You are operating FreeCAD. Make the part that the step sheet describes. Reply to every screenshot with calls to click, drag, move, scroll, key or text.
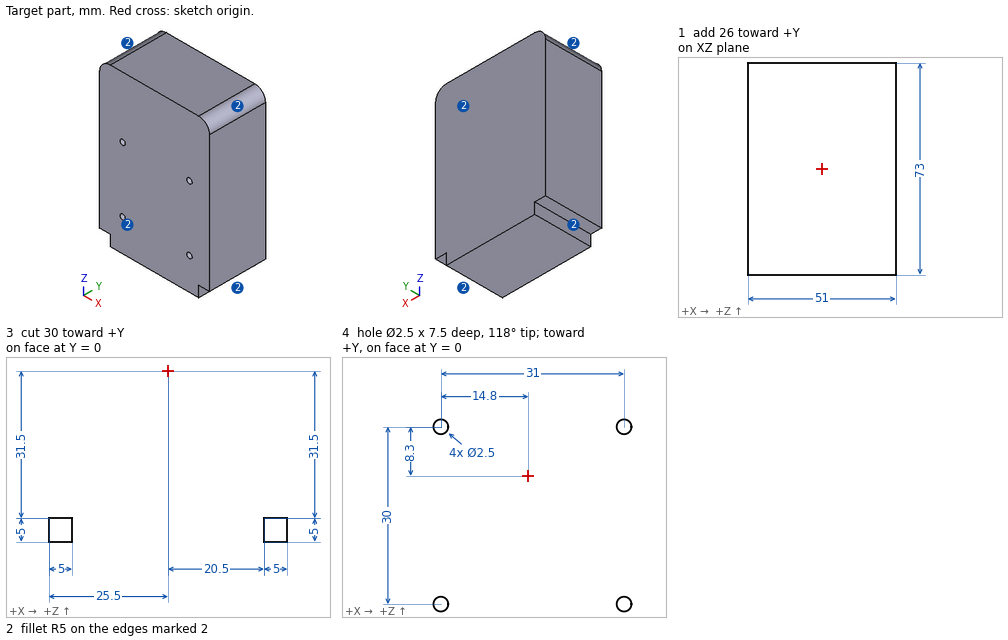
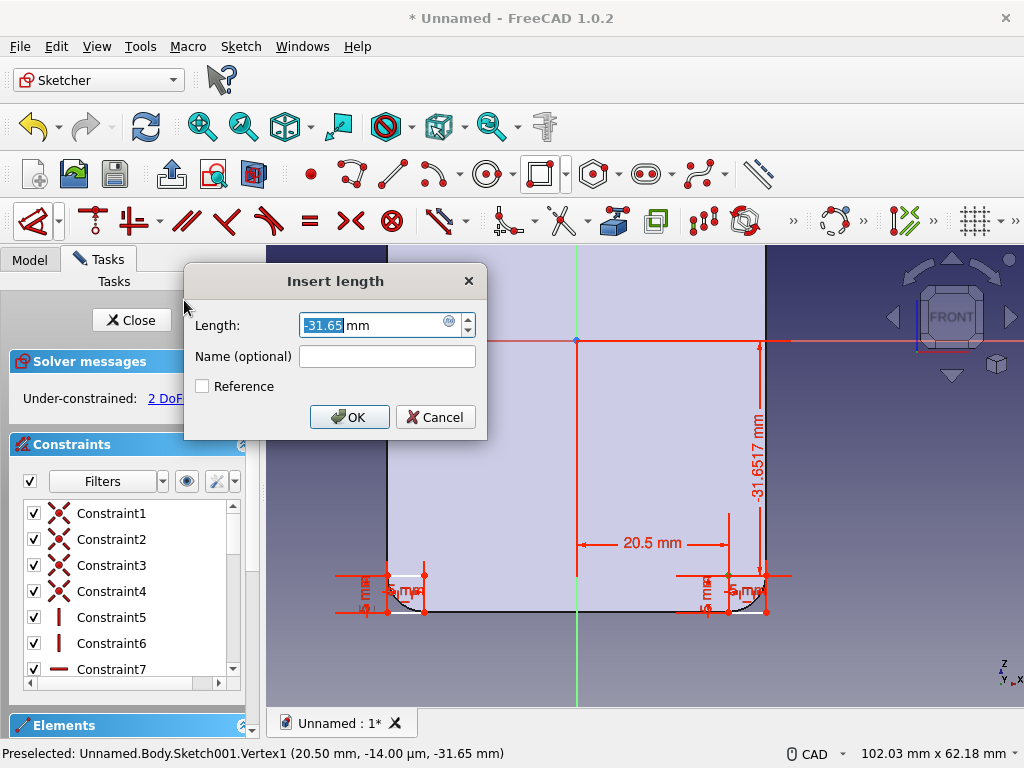
text(-31.5)
key(Return)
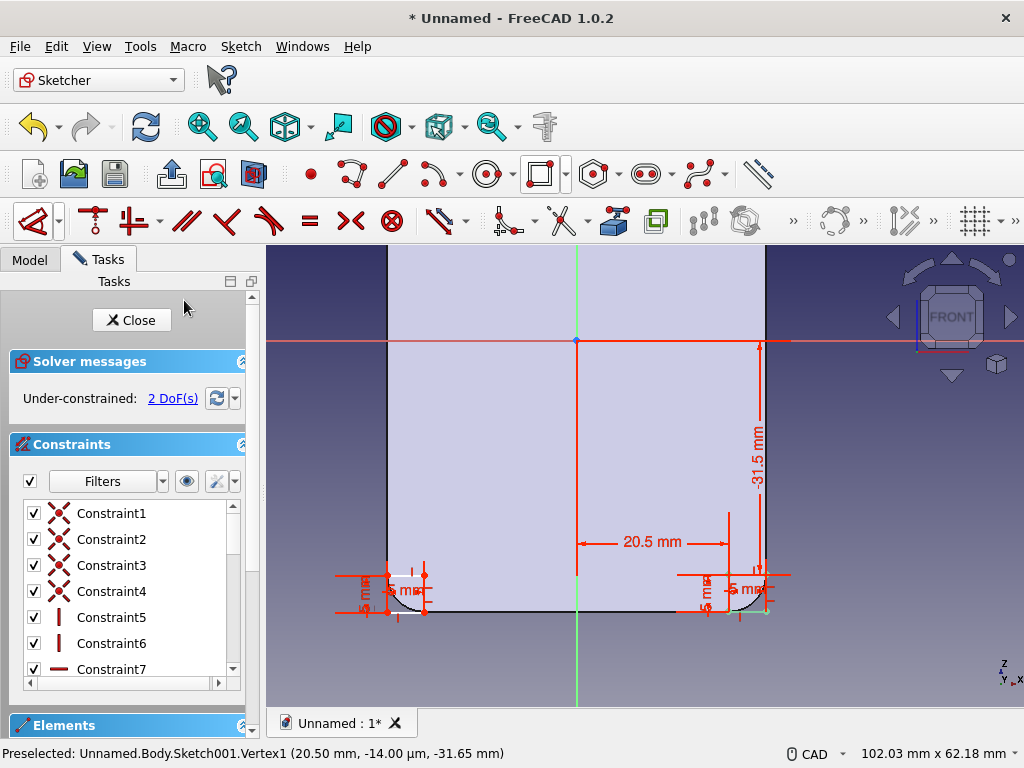
click(387, 576)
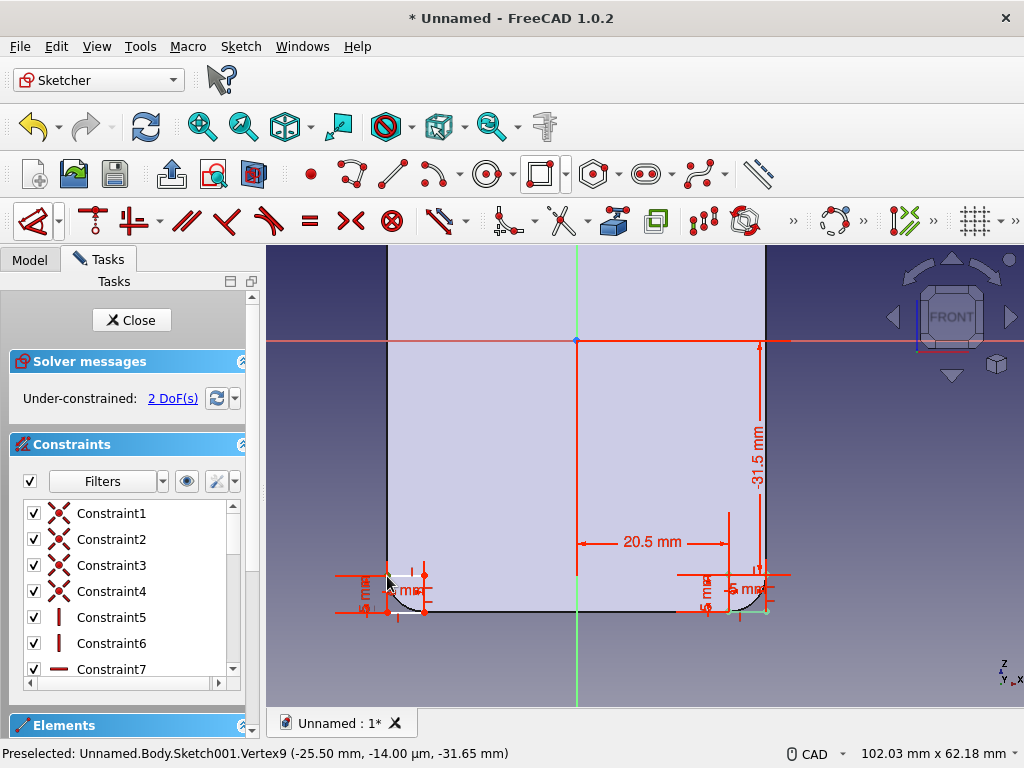
click(58, 222)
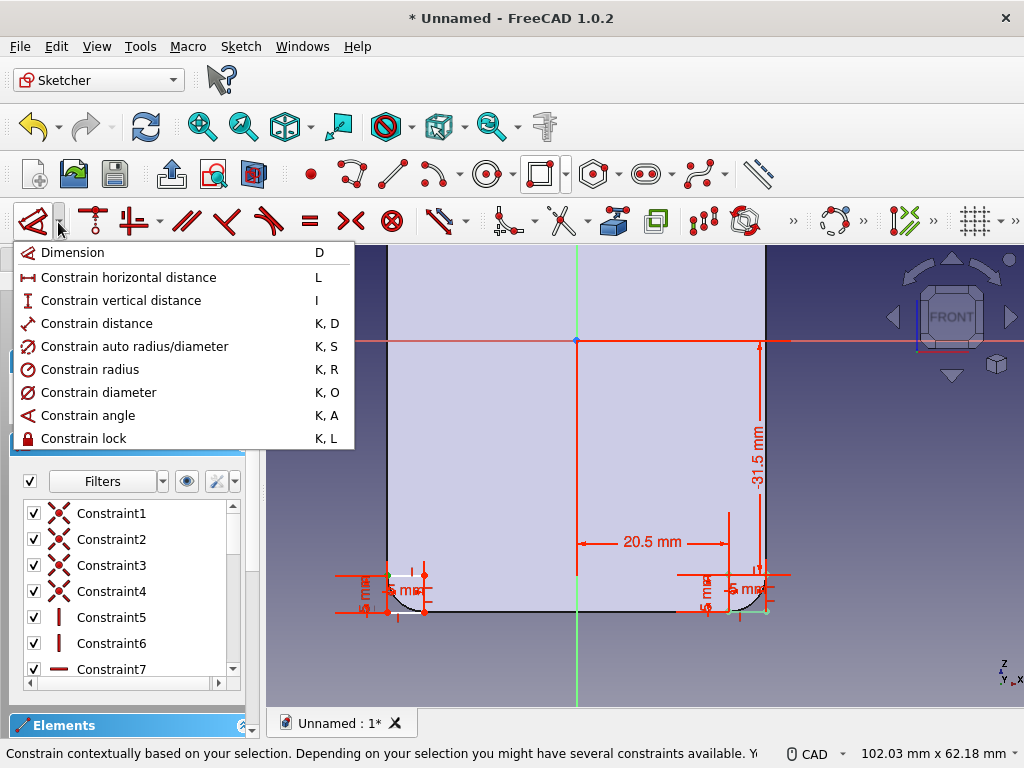
click(184, 278)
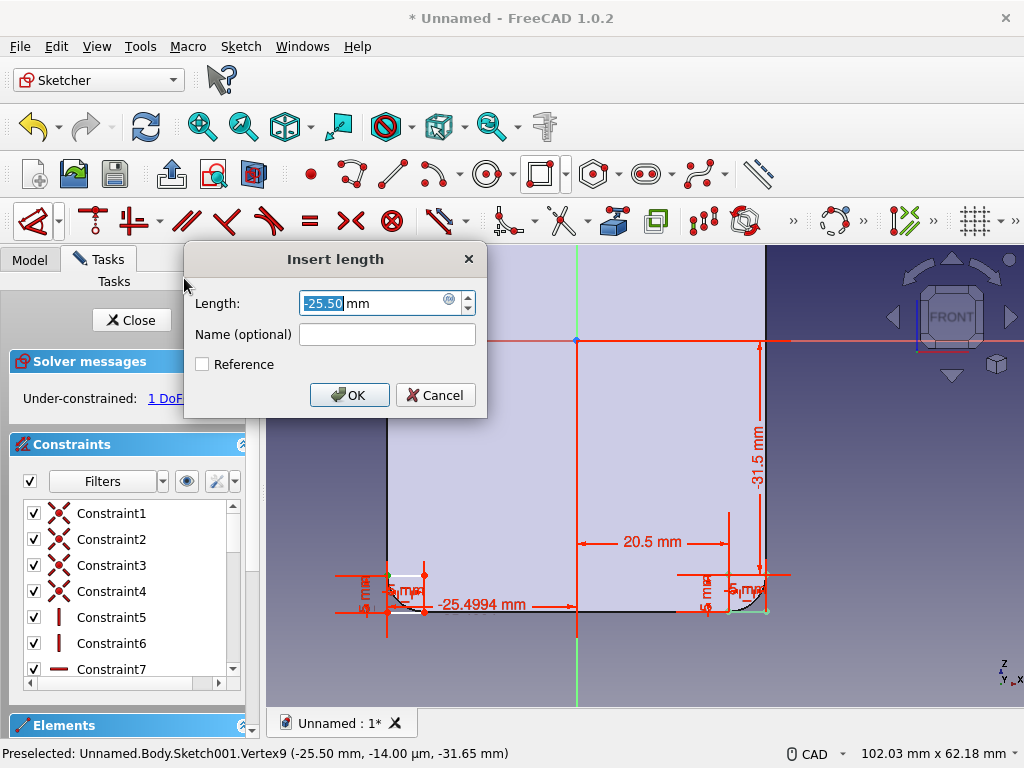
text(-25.5)
key(Return)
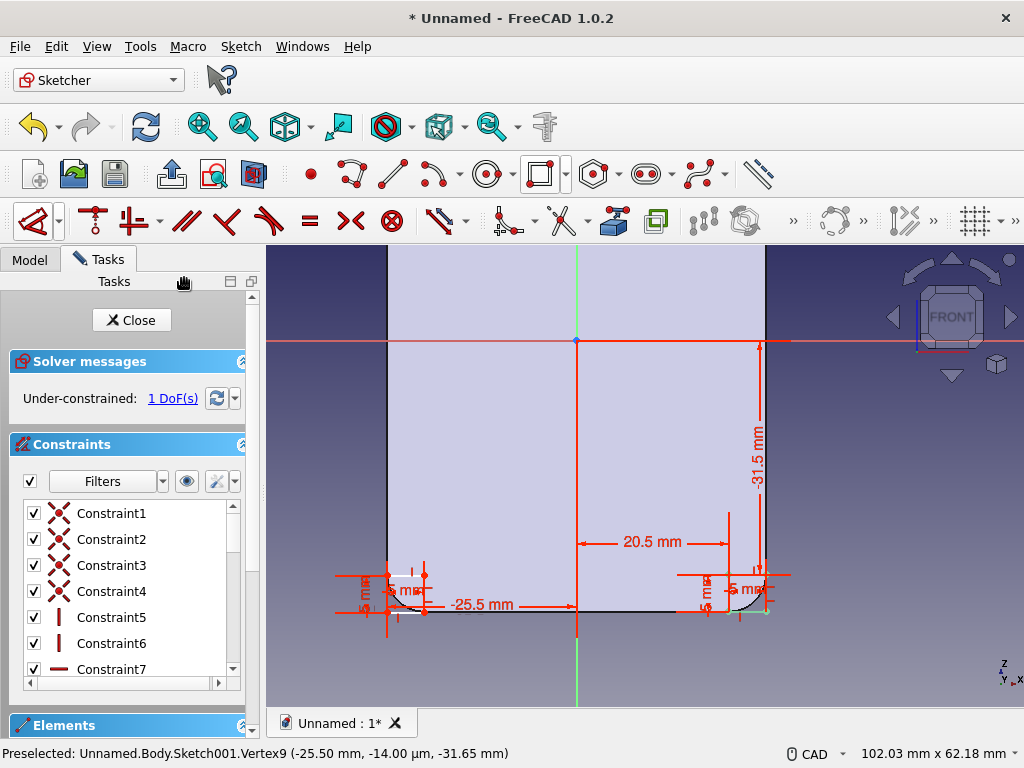
click(387, 576)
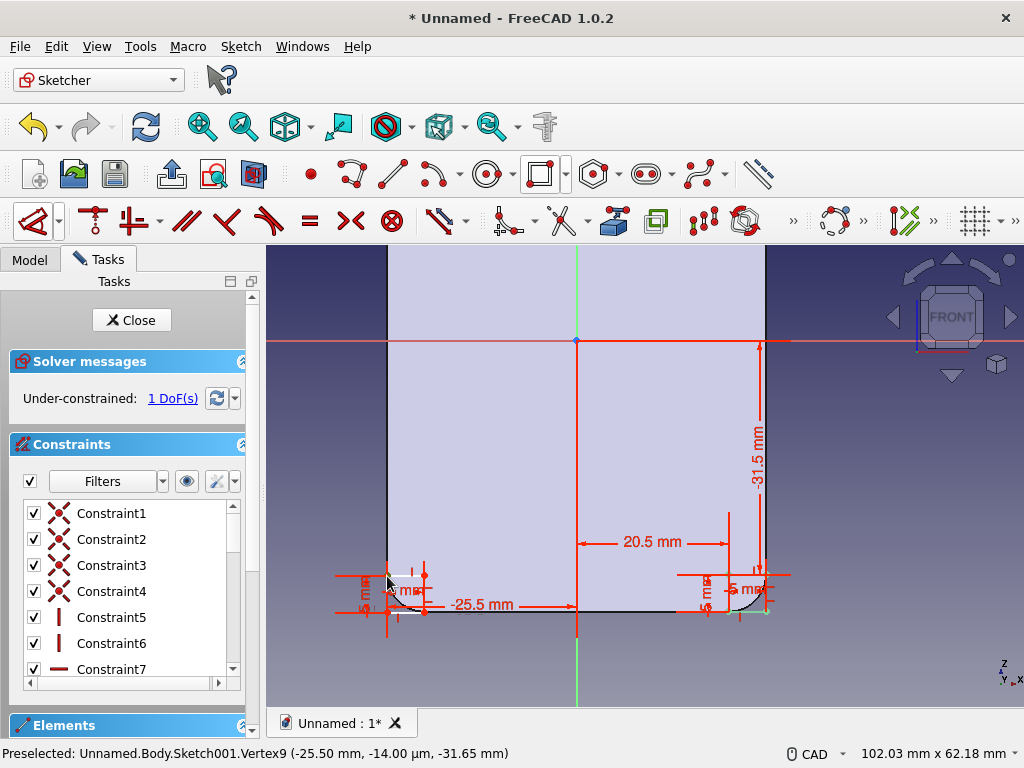
key(i)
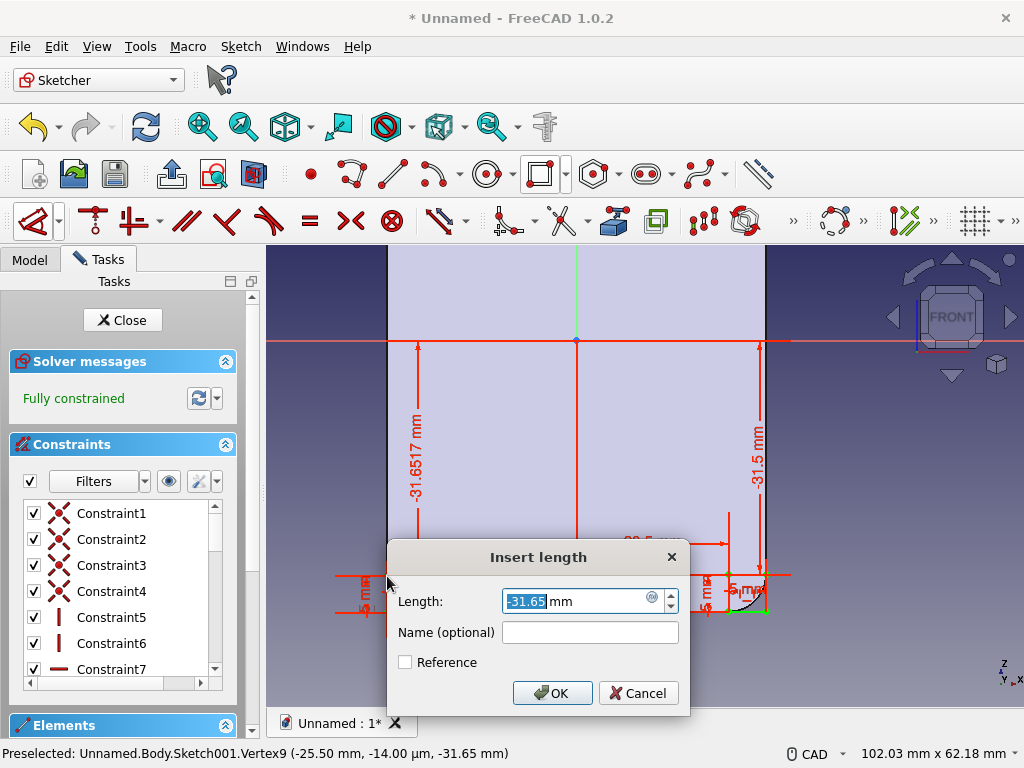
text(-31.5)
key(Return)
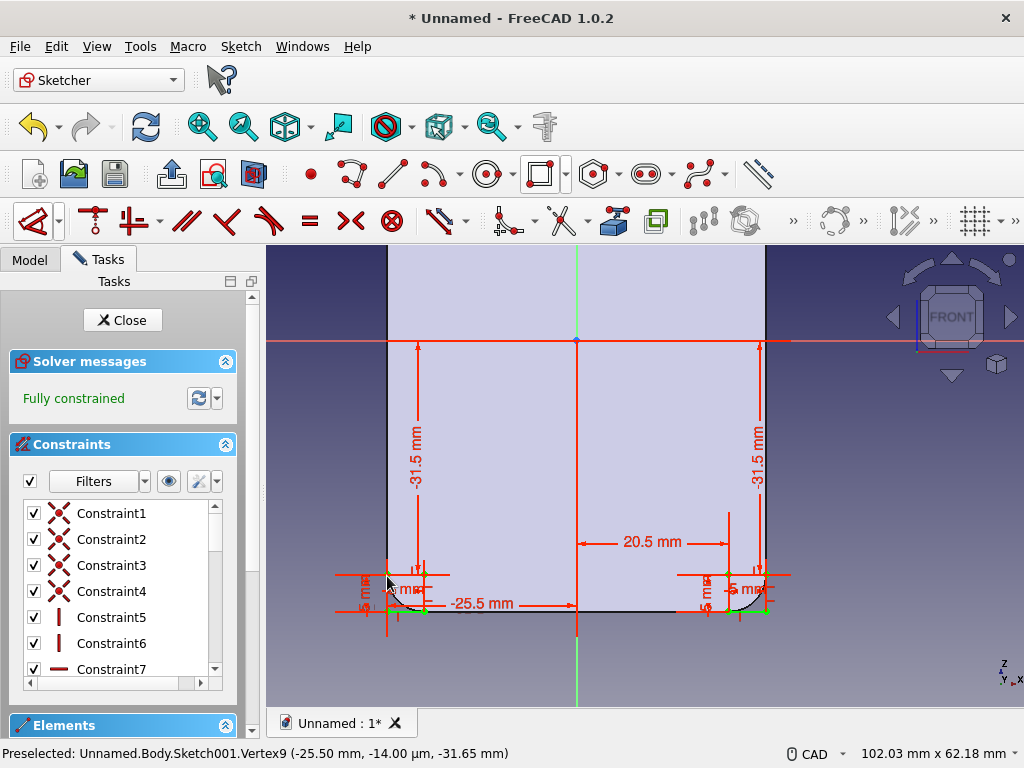
click(123, 320)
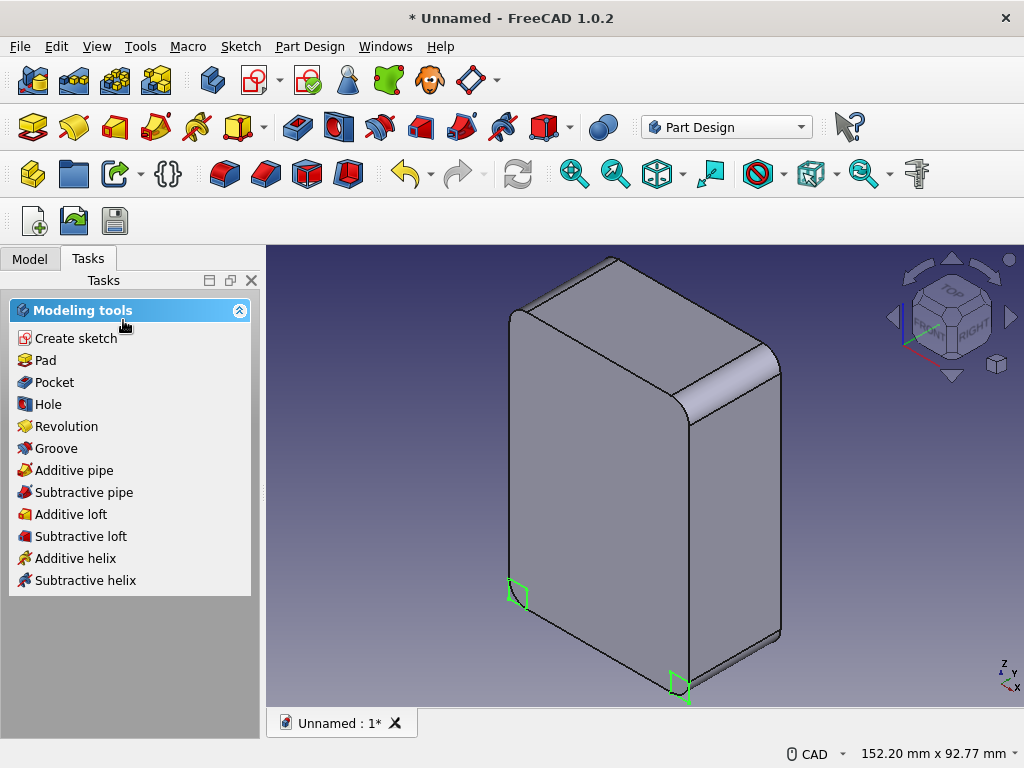
click(298, 128)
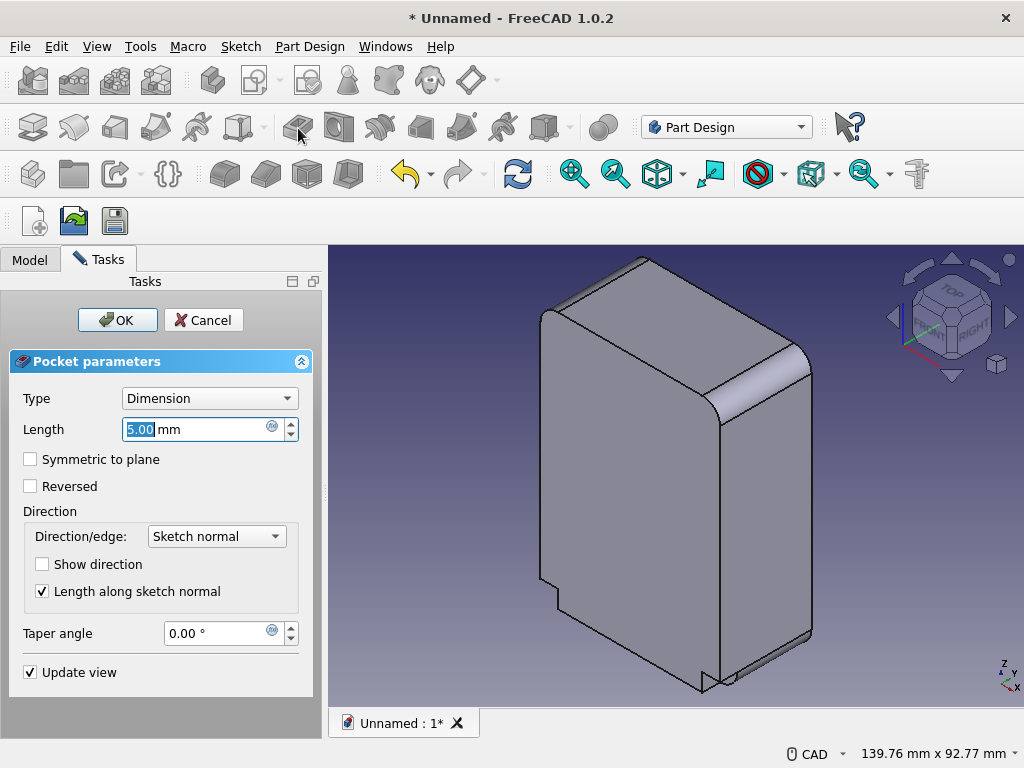
text(30)
key(Tab)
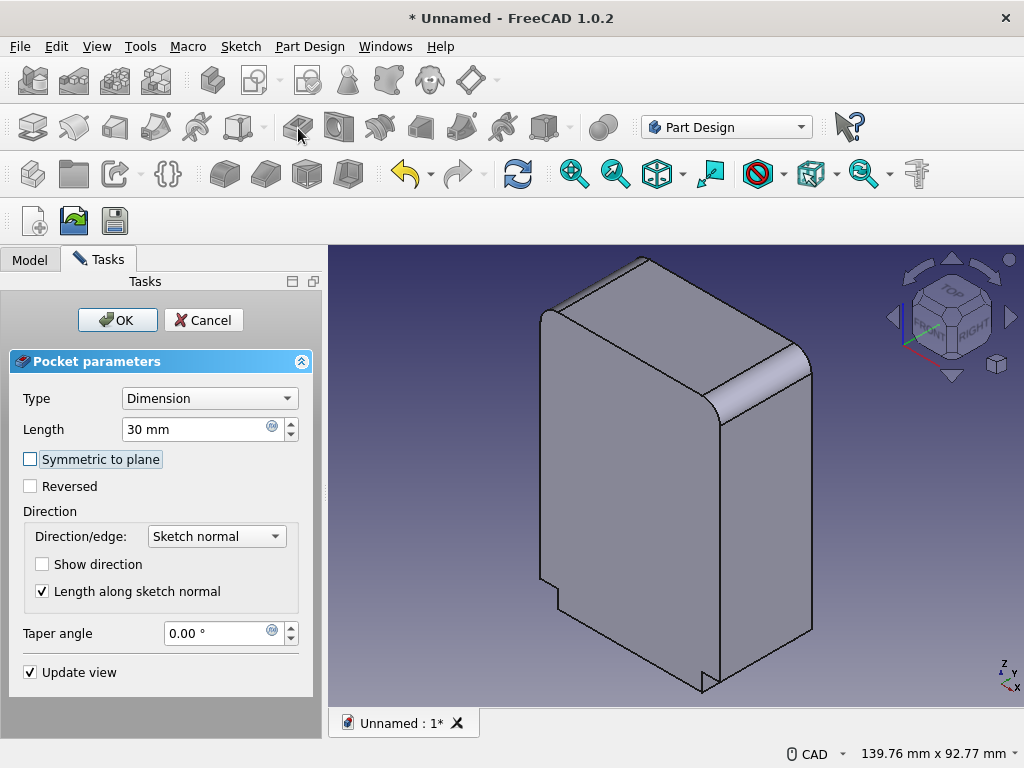
click(118, 320)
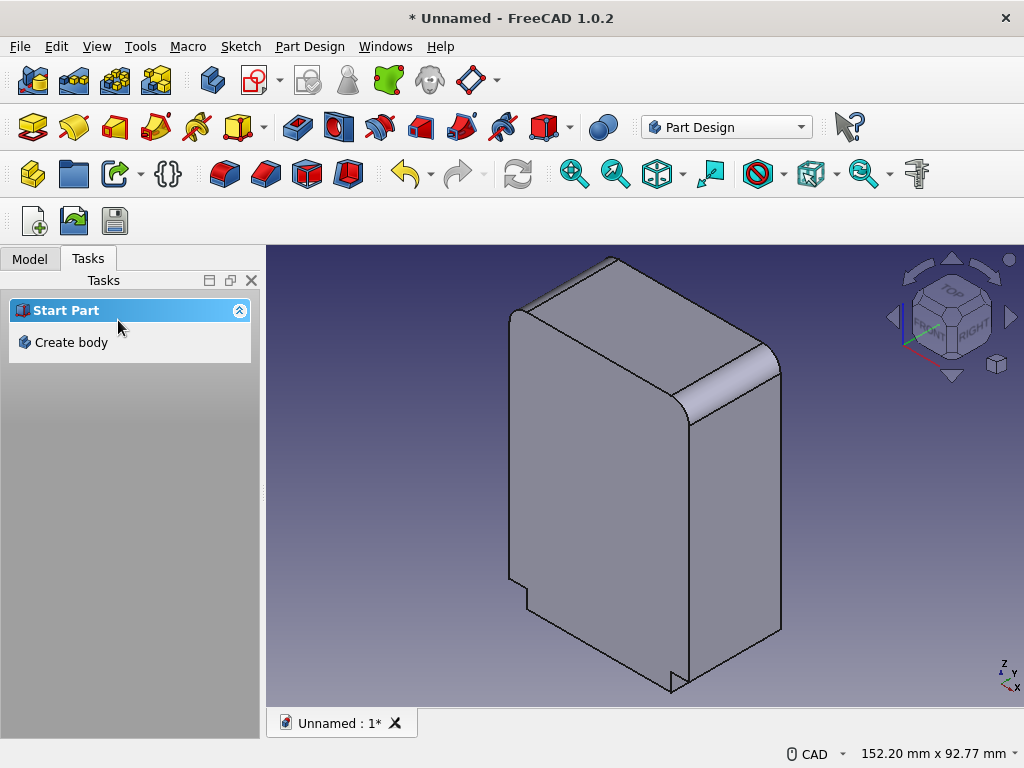
click(599, 459)